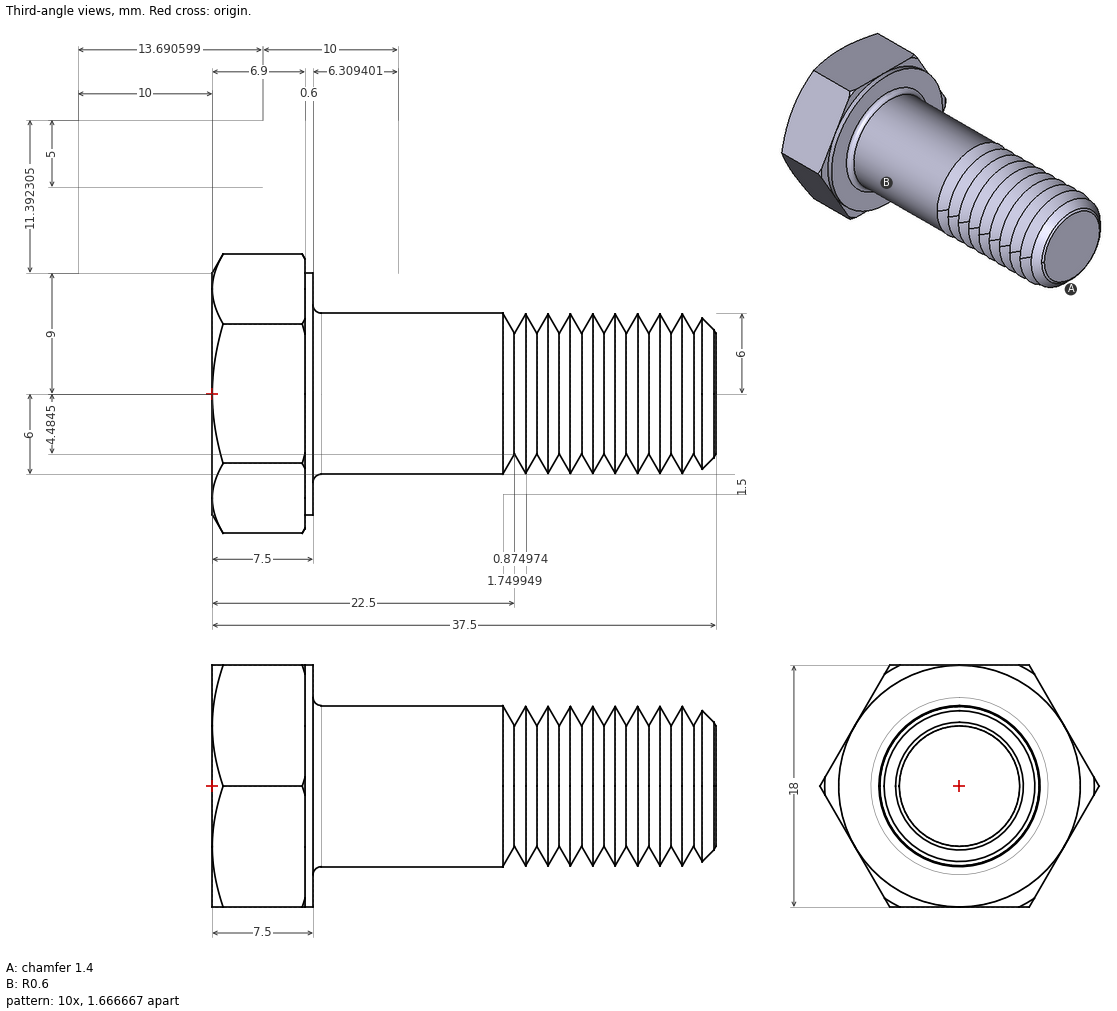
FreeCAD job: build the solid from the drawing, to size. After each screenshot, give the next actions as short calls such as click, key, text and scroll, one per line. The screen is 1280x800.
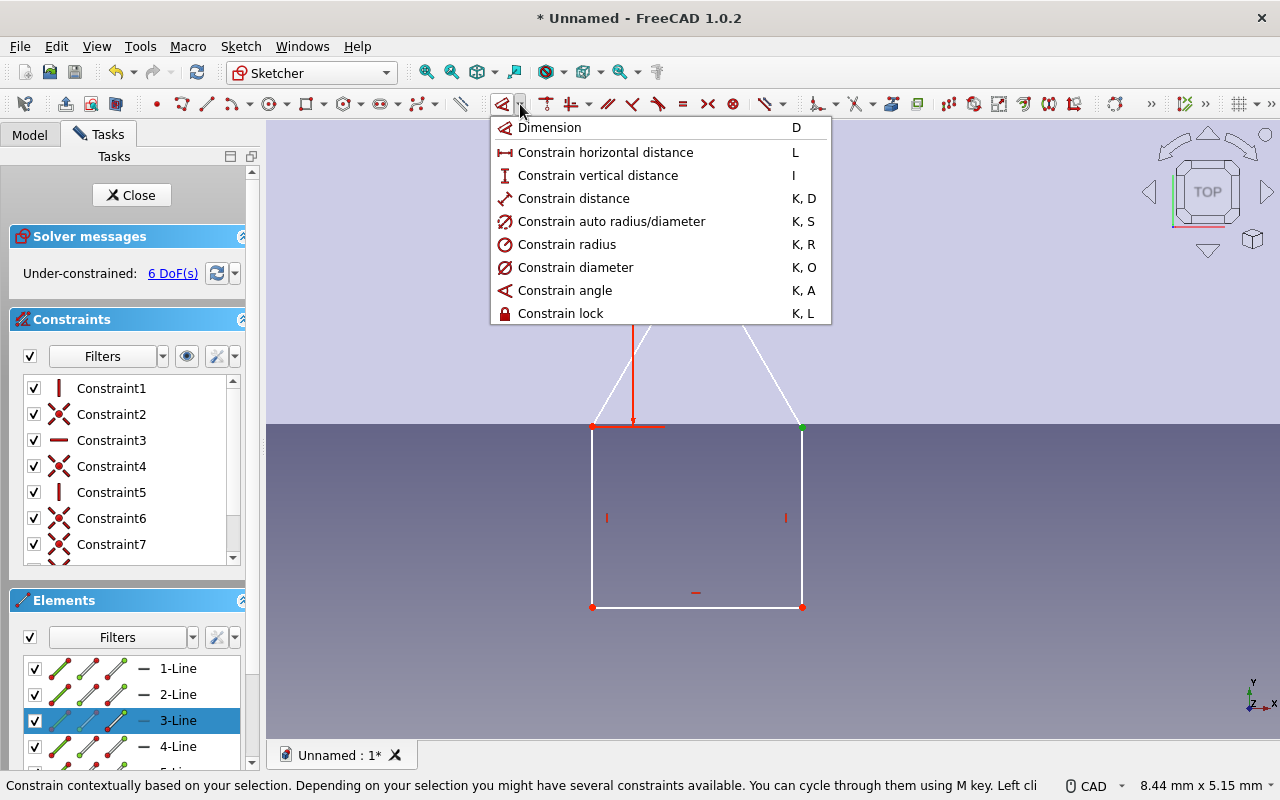
click(661, 176)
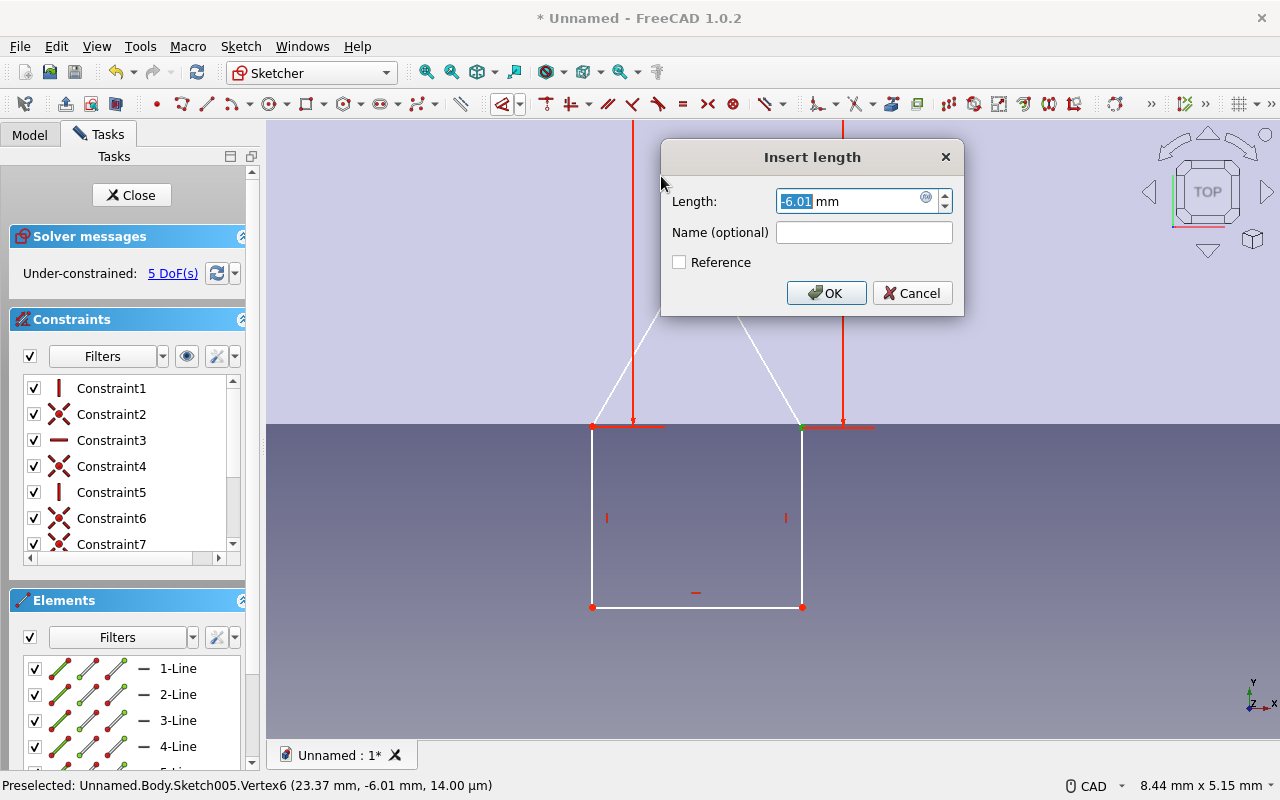
text(-6)
key(Return)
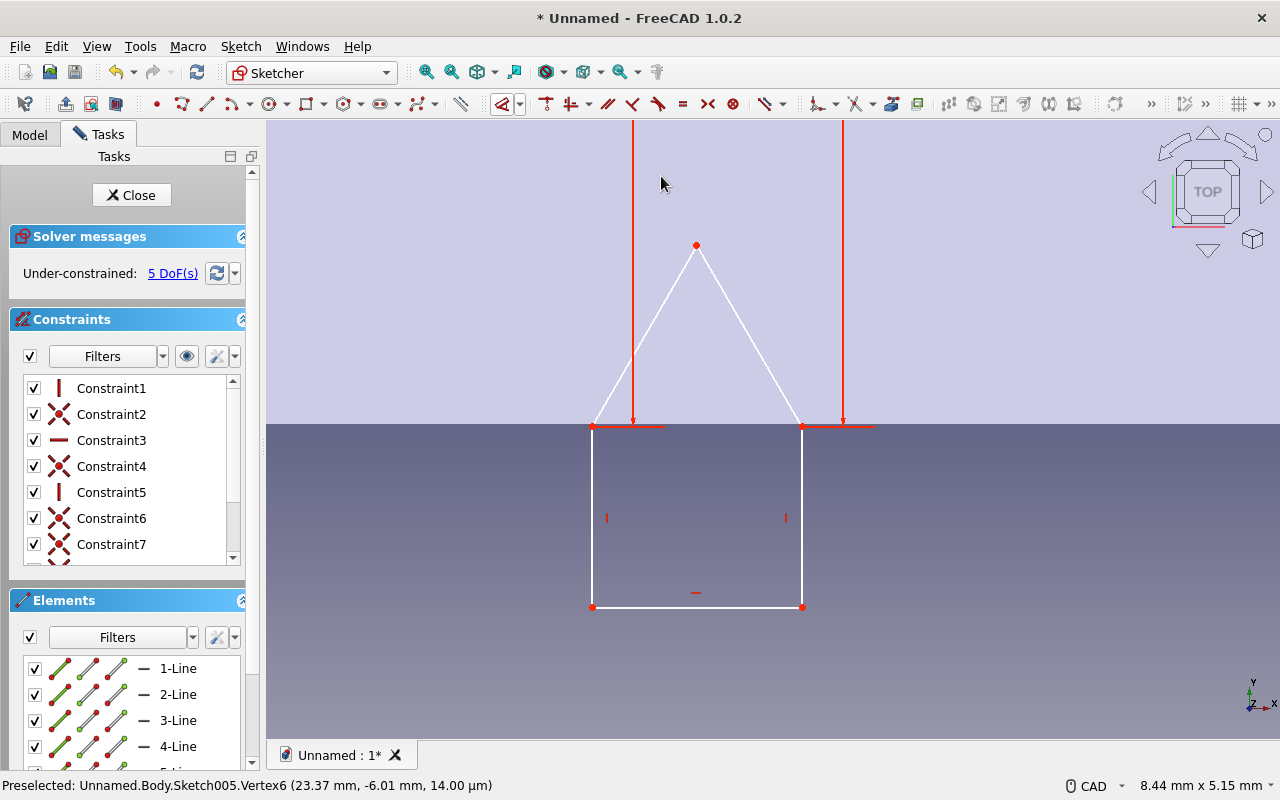
click(592, 481)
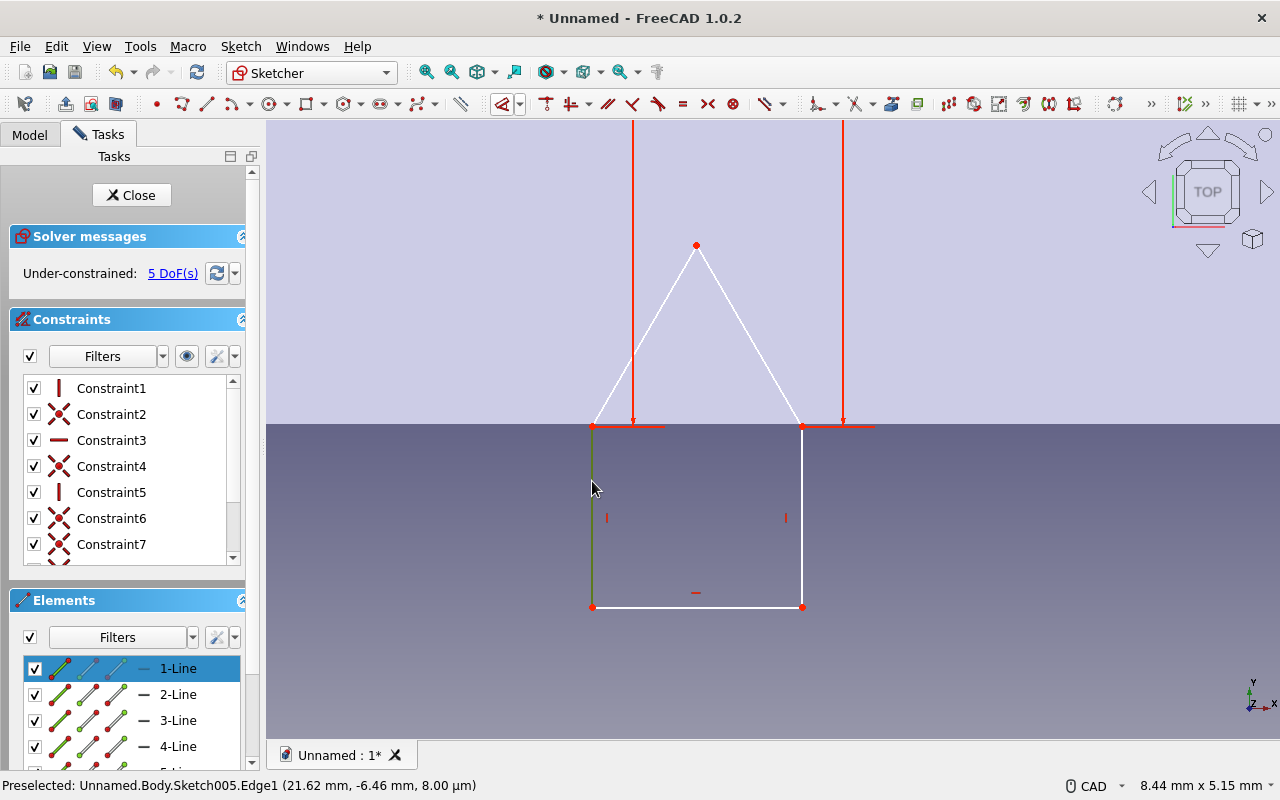
key(i)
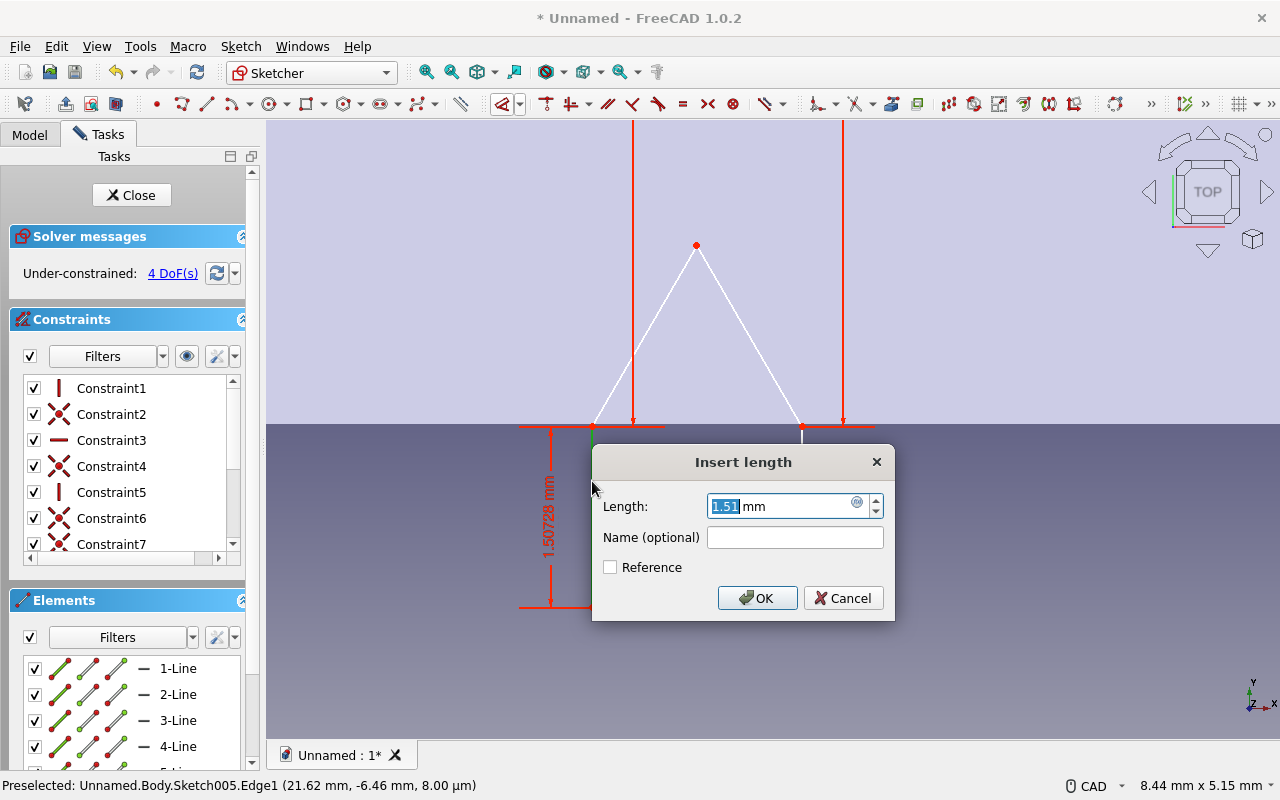
text(1.5)
key(Return)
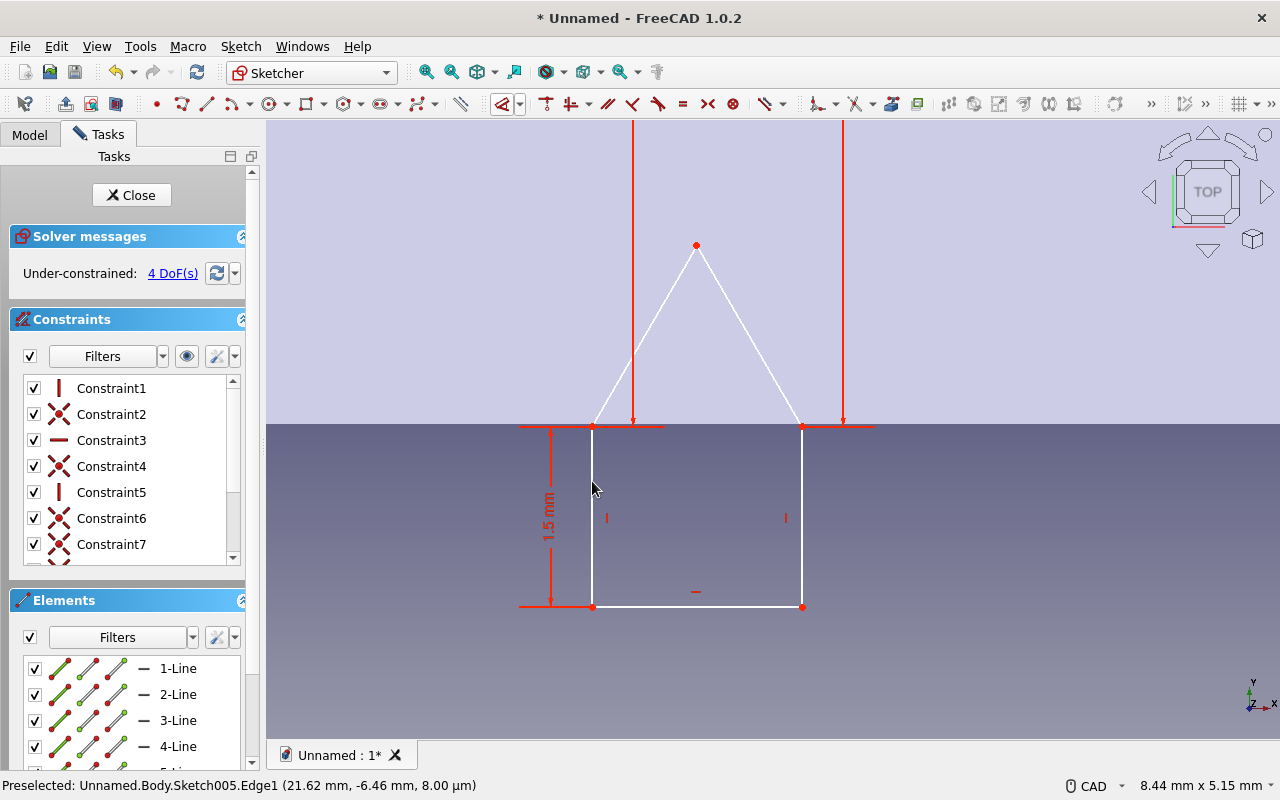
click(697, 246)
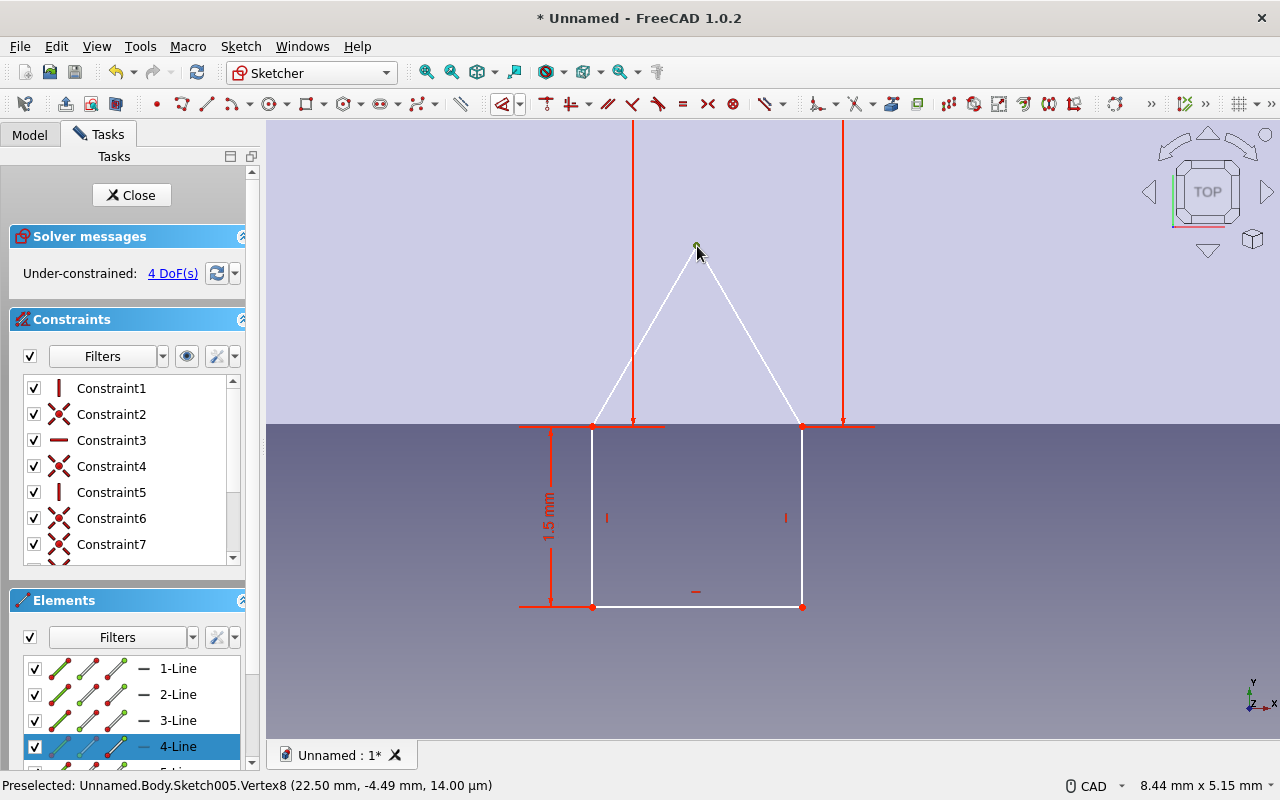
key(l)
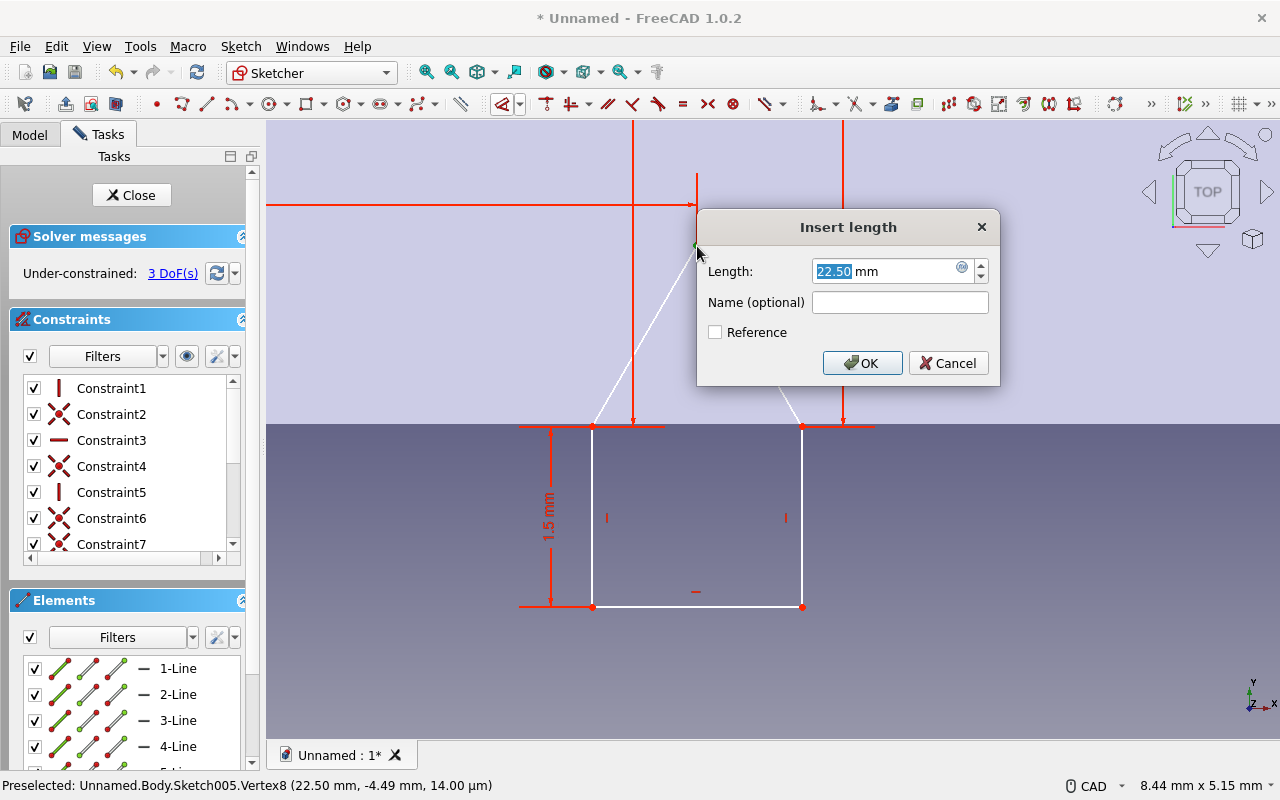
text(22.5)
key(Return)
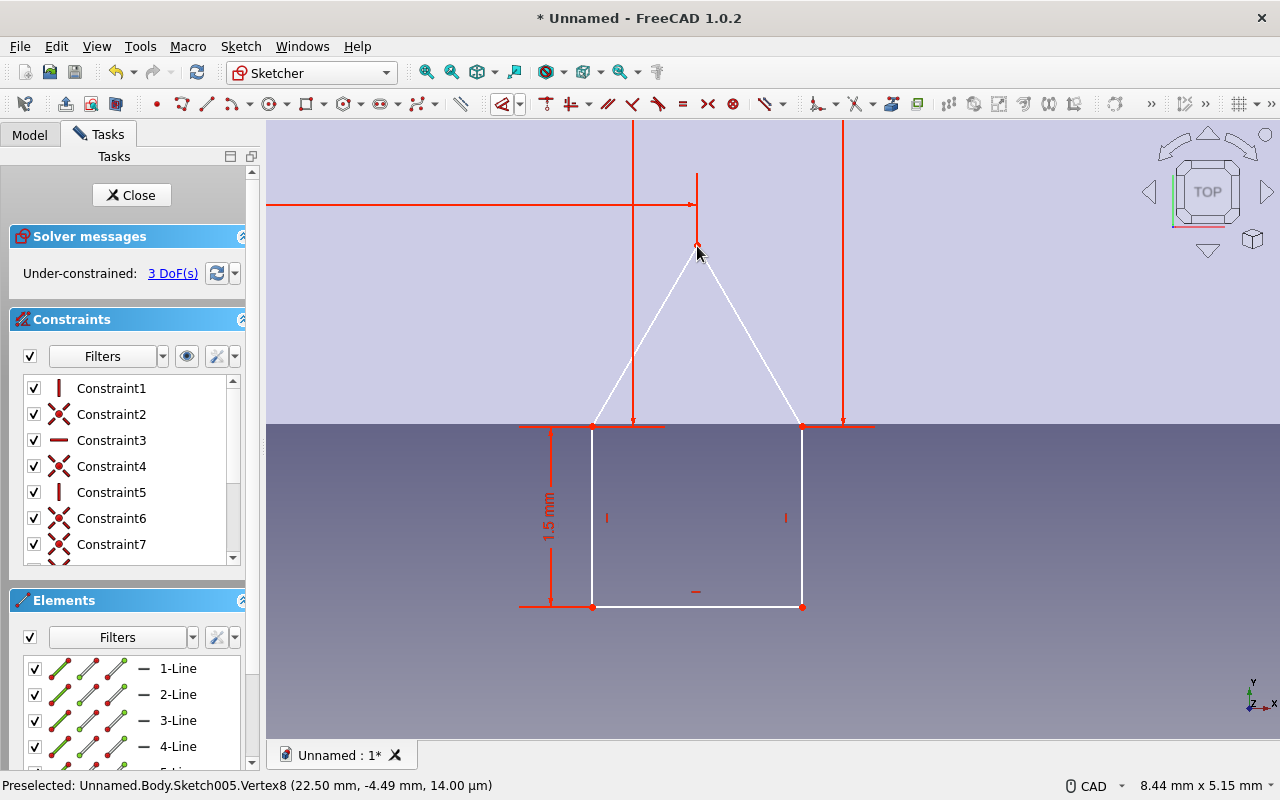
click(697, 246)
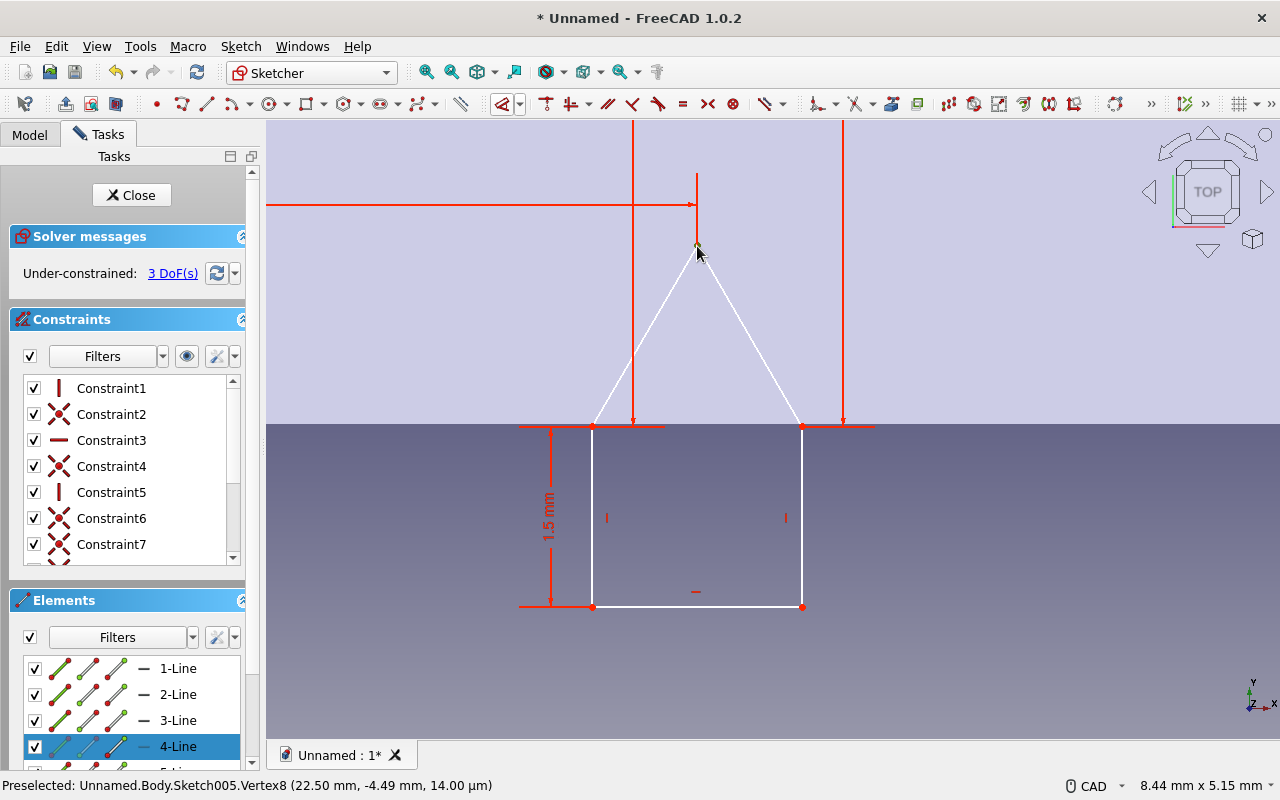
click(520, 104)